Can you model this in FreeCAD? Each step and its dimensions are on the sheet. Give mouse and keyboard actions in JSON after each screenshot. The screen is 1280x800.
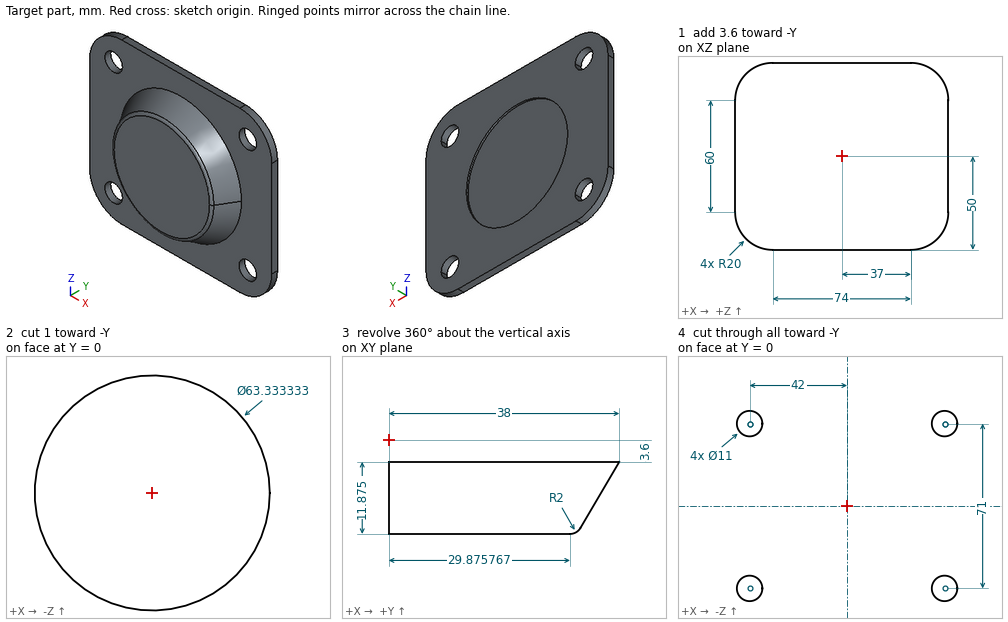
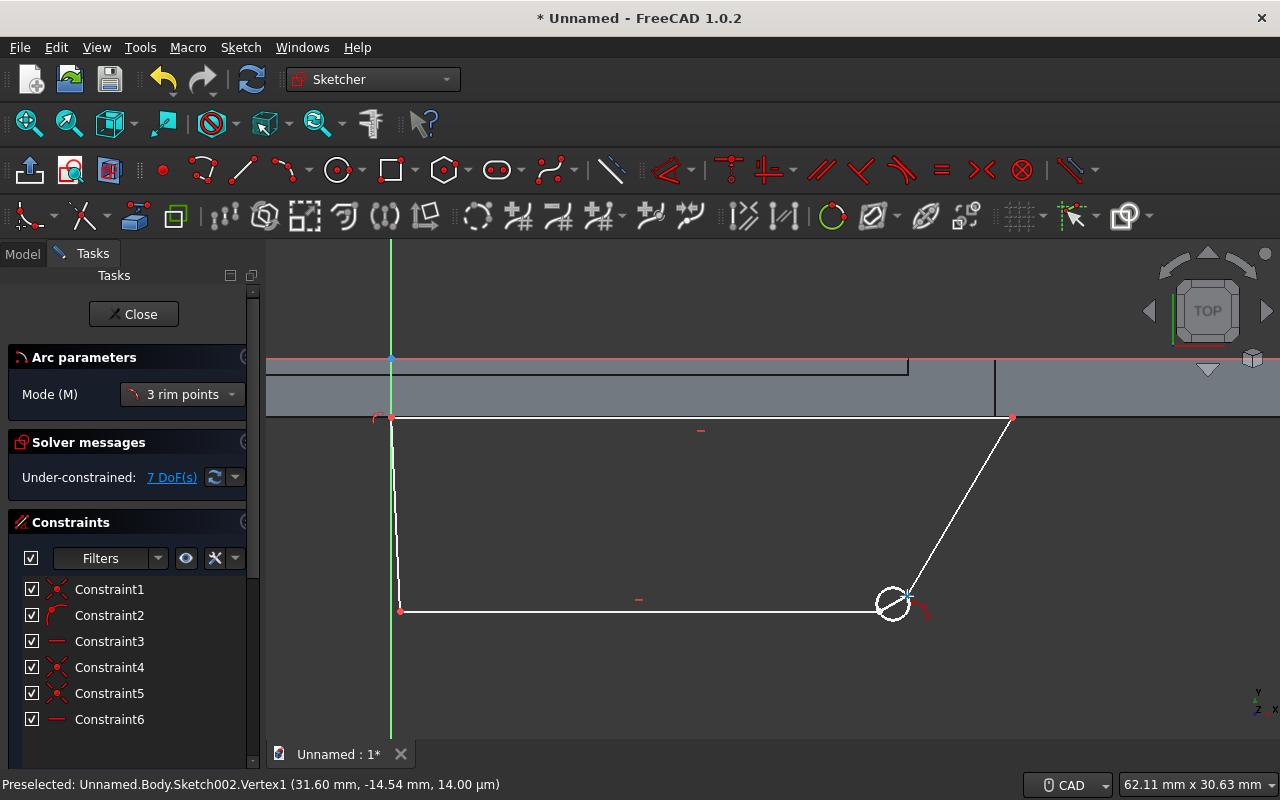
{"action": "scroll", "coordinate": [895, 607], "scroll_direction": "up", "scroll_amount": 7}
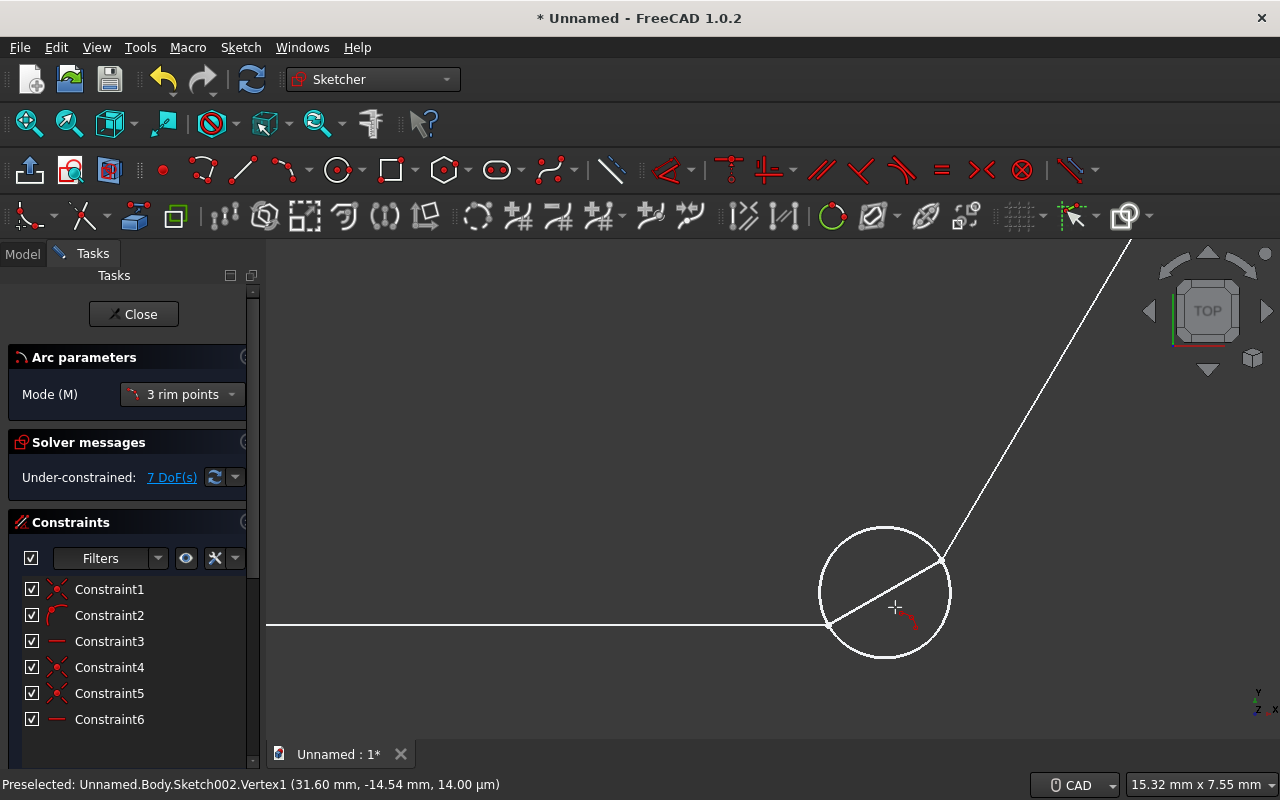
{"action": "left_click", "coordinate": [894, 605]}
{"action": "key", "text": "Escape"}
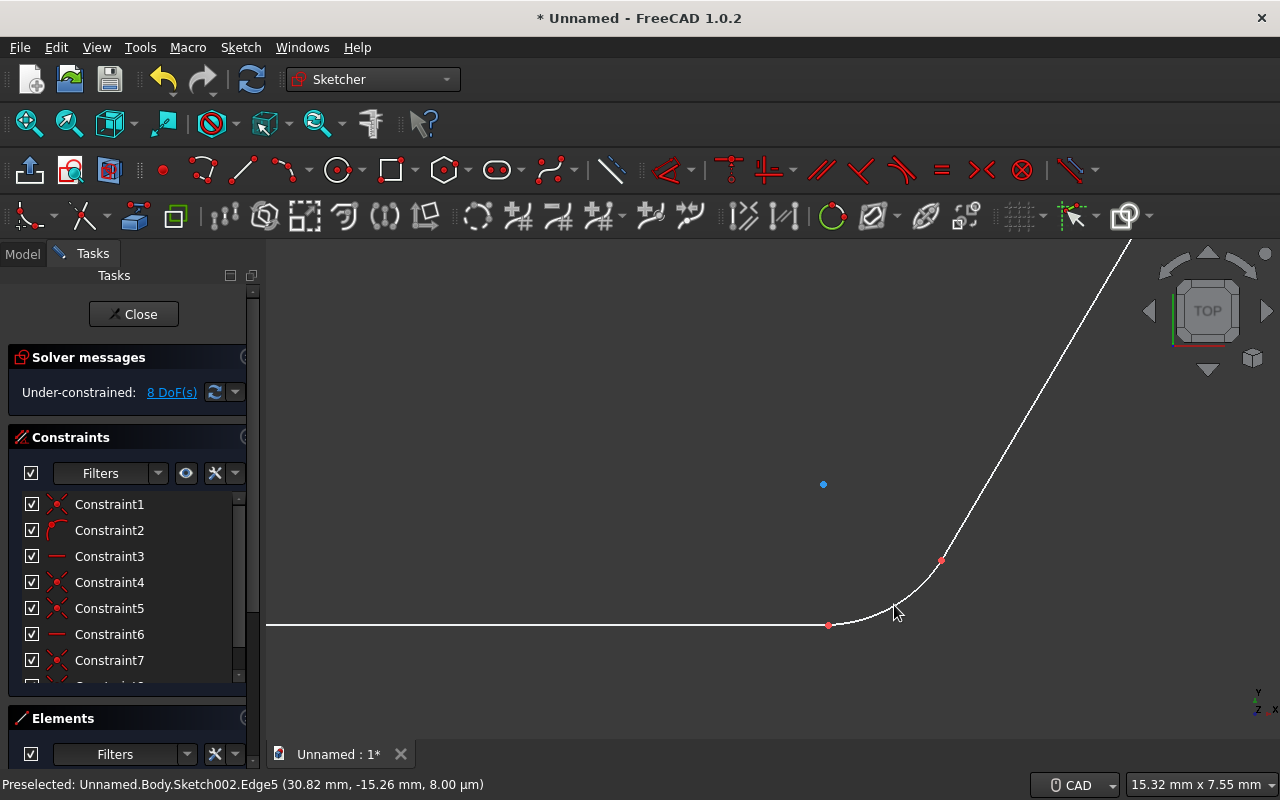
{"action": "scroll", "coordinate": [900, 613], "scroll_direction": "down", "scroll_amount": 7}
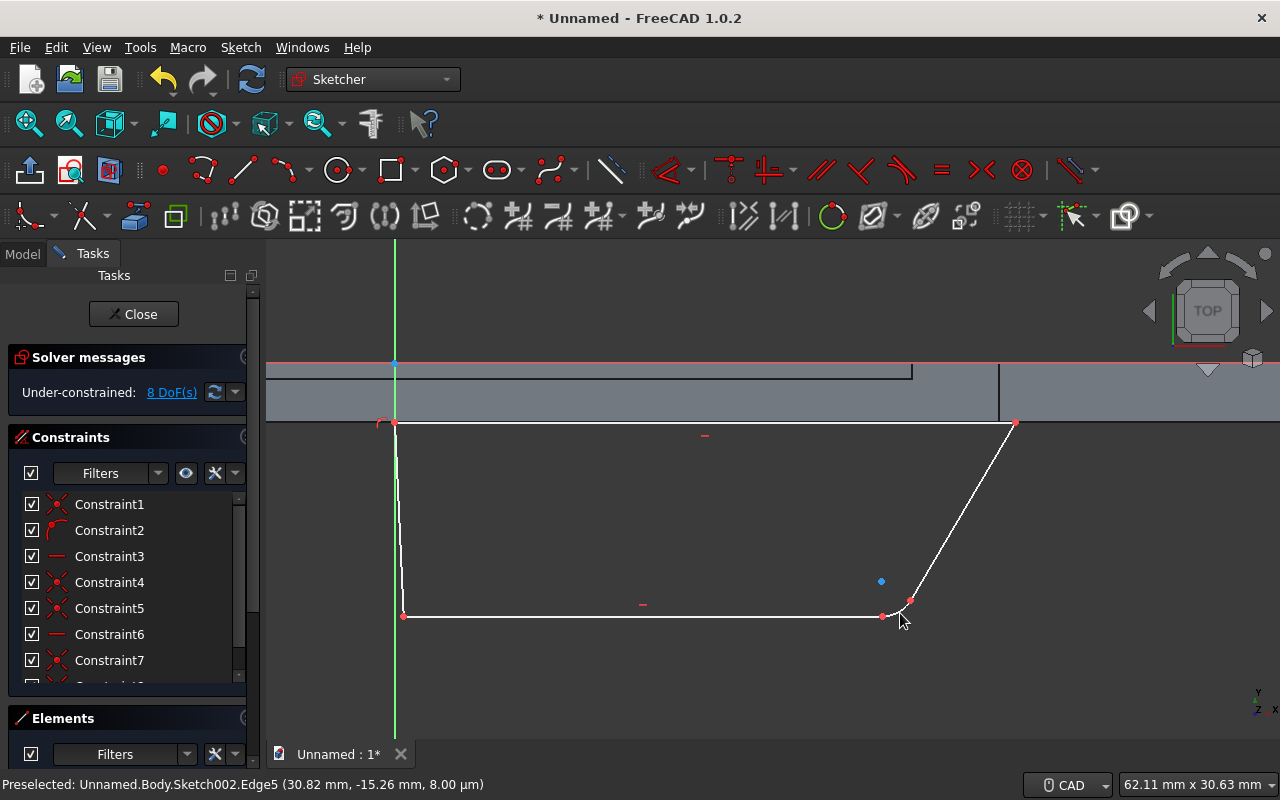
{"action": "left_click", "coordinate": [942, 547]}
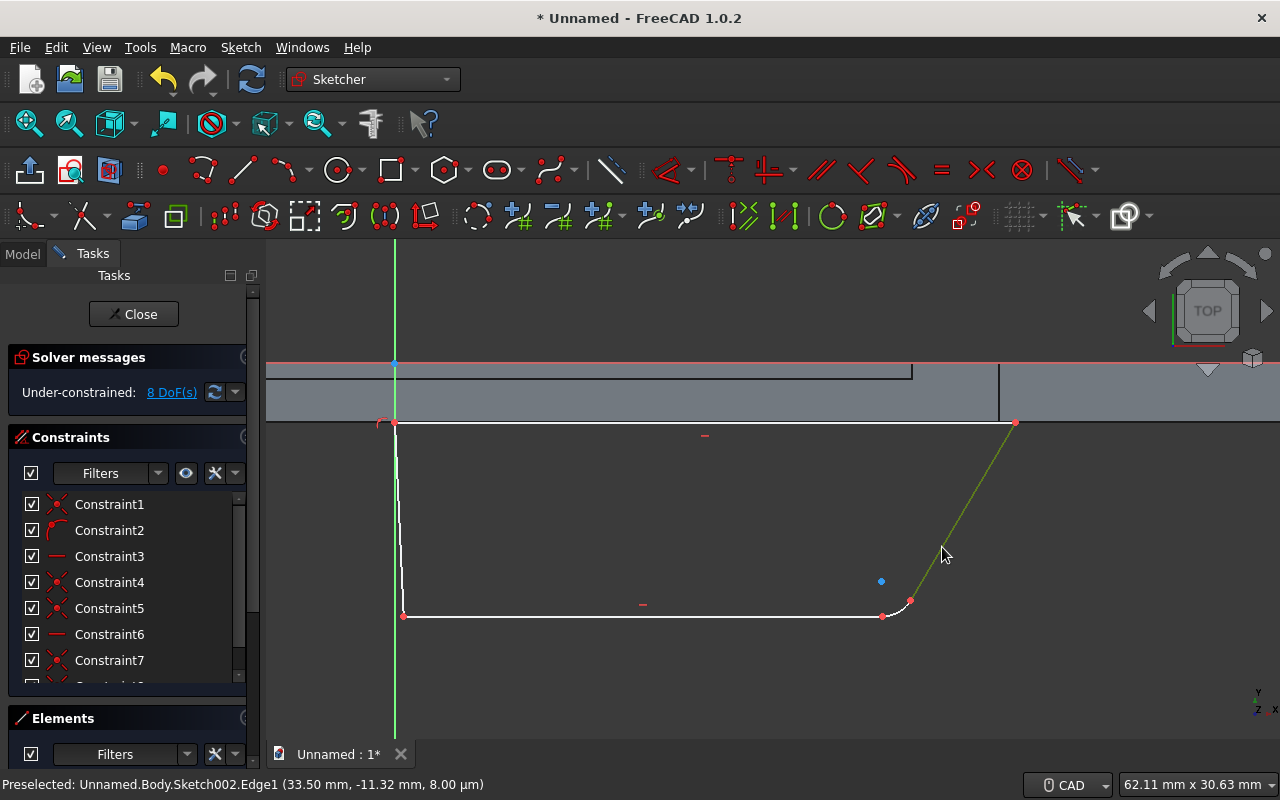
{"action": "scroll", "coordinate": [893, 615], "scroll_direction": "up", "scroll_amount": 2}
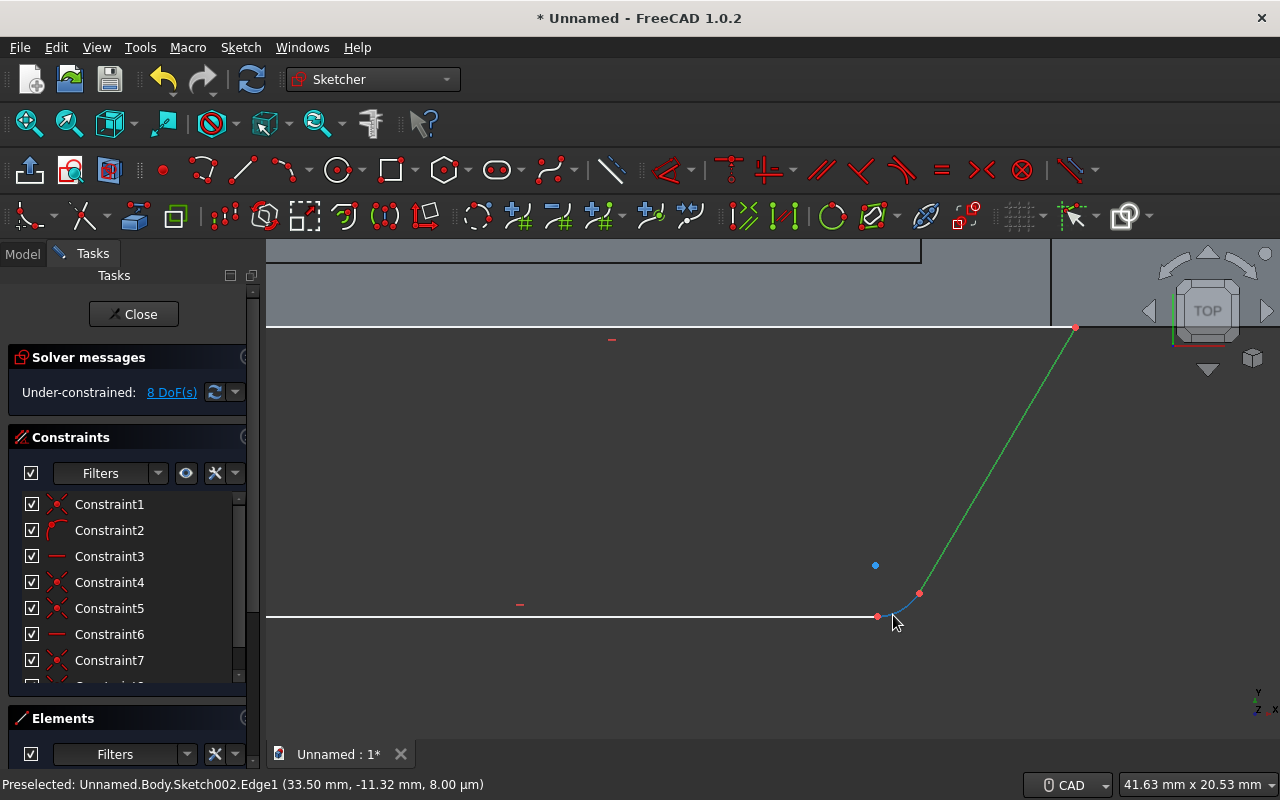
{"action": "left_click", "coordinate": [892, 614]}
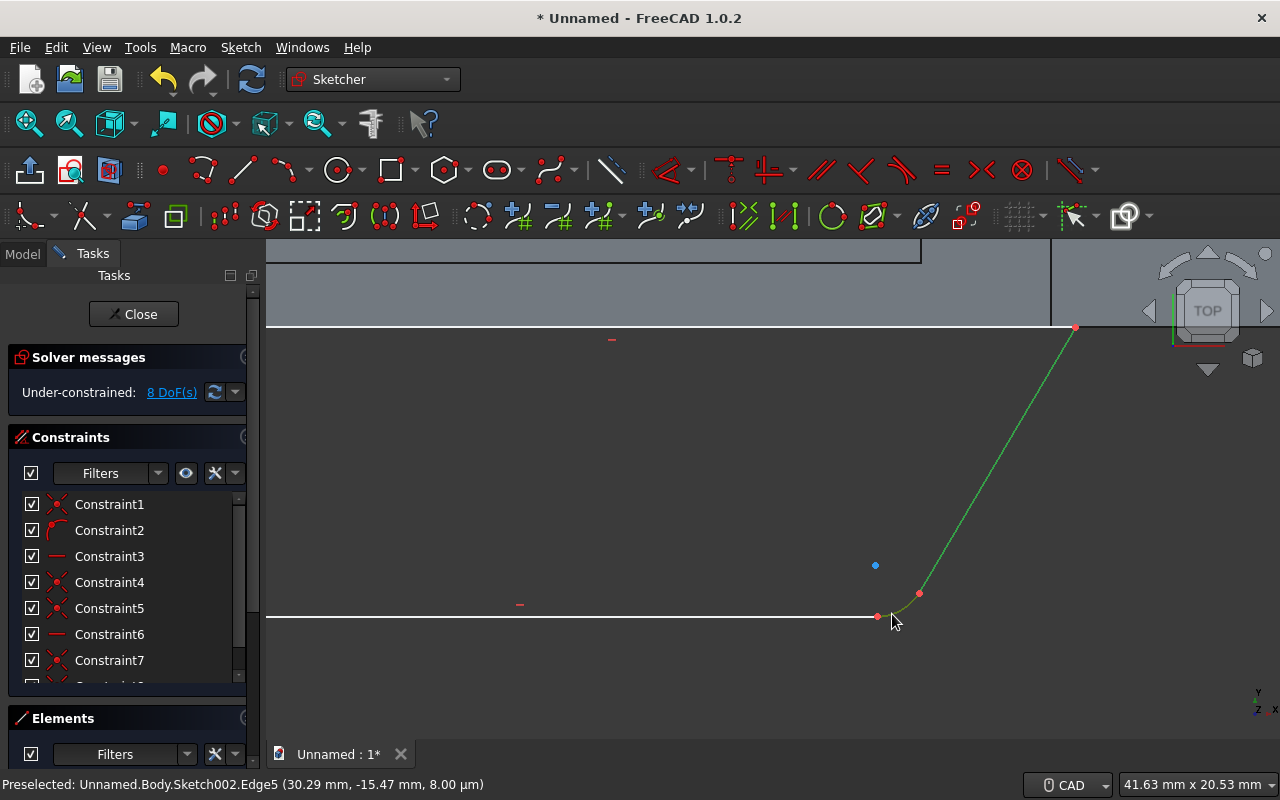
{"action": "left_click", "coordinate": [902, 170]}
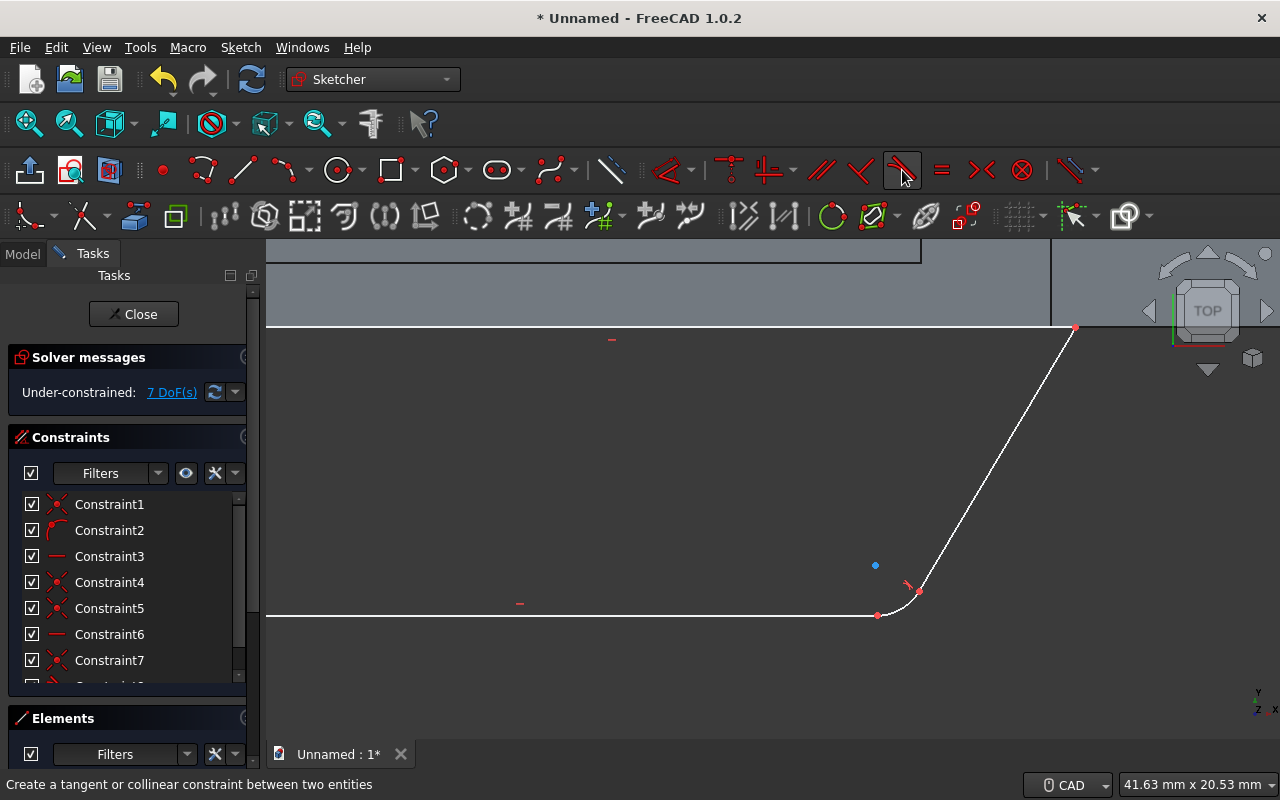
{"action": "left_click", "coordinate": [377, 616]}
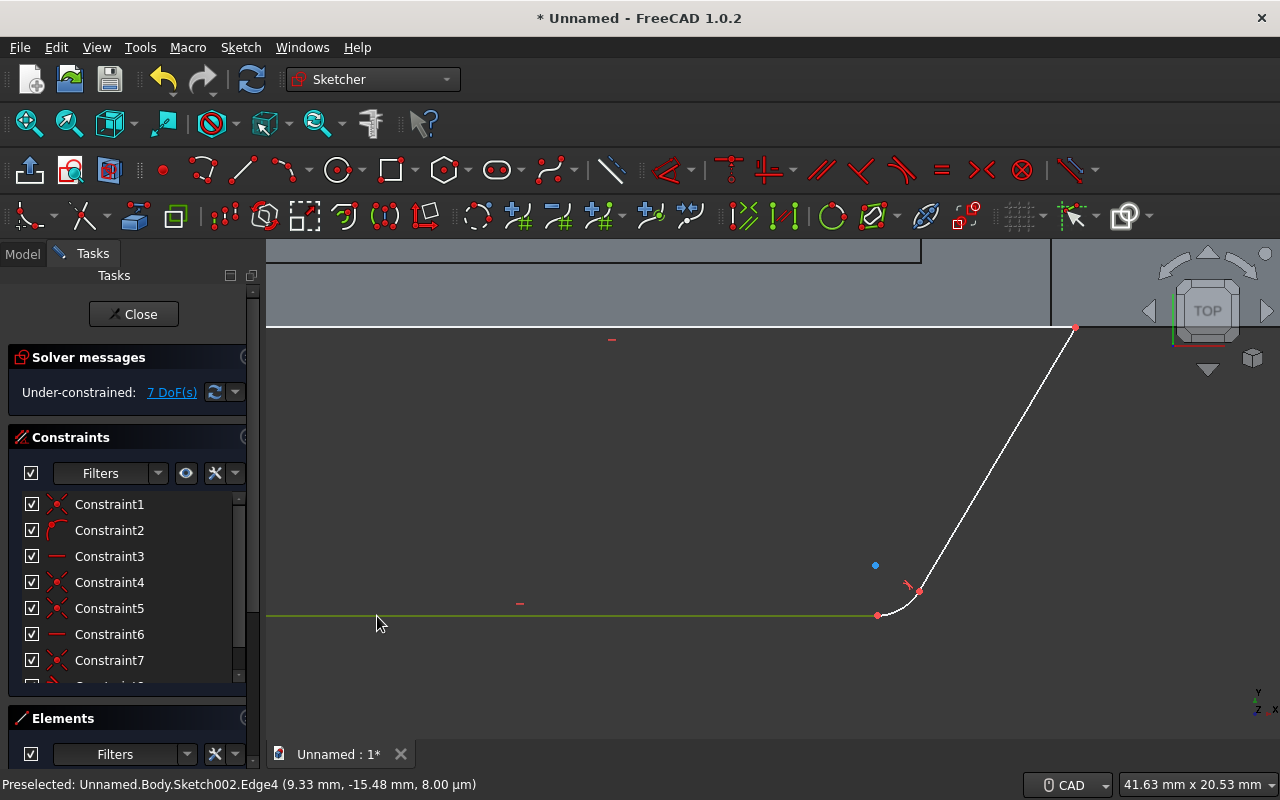
{"action": "left_click", "coordinate": [892, 613]}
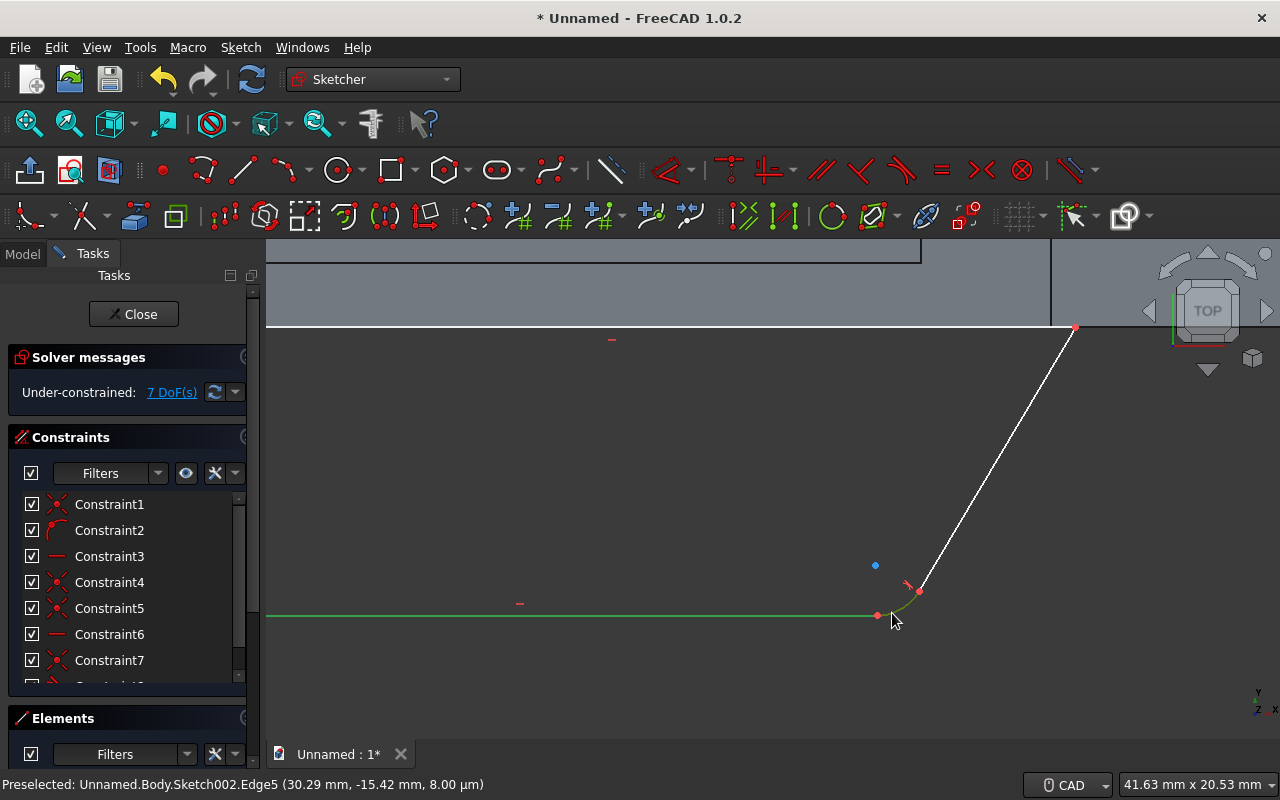
{"action": "left_click", "coordinate": [902, 170]}